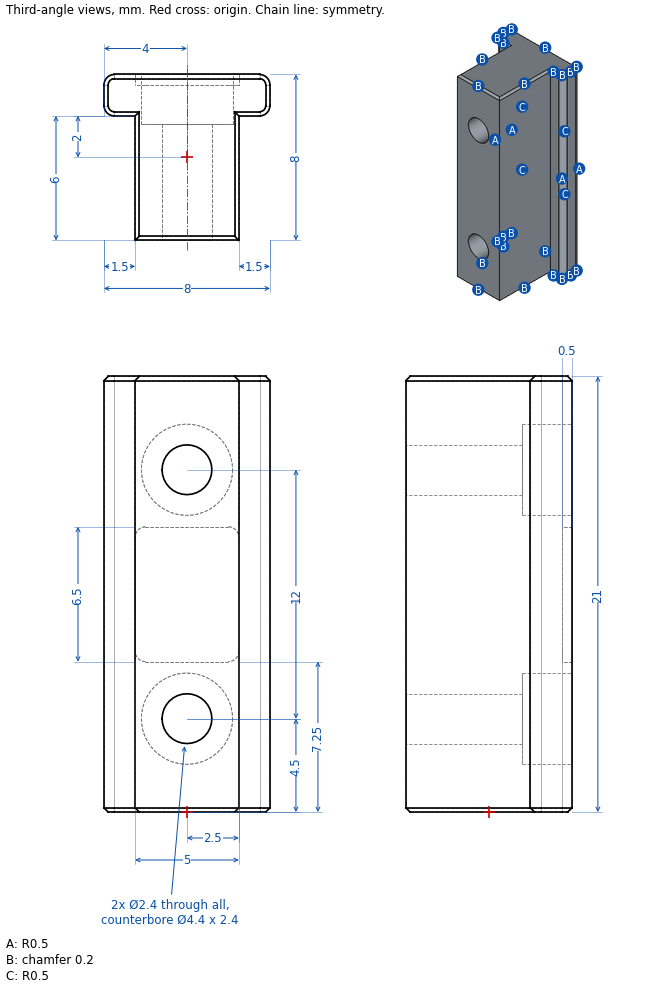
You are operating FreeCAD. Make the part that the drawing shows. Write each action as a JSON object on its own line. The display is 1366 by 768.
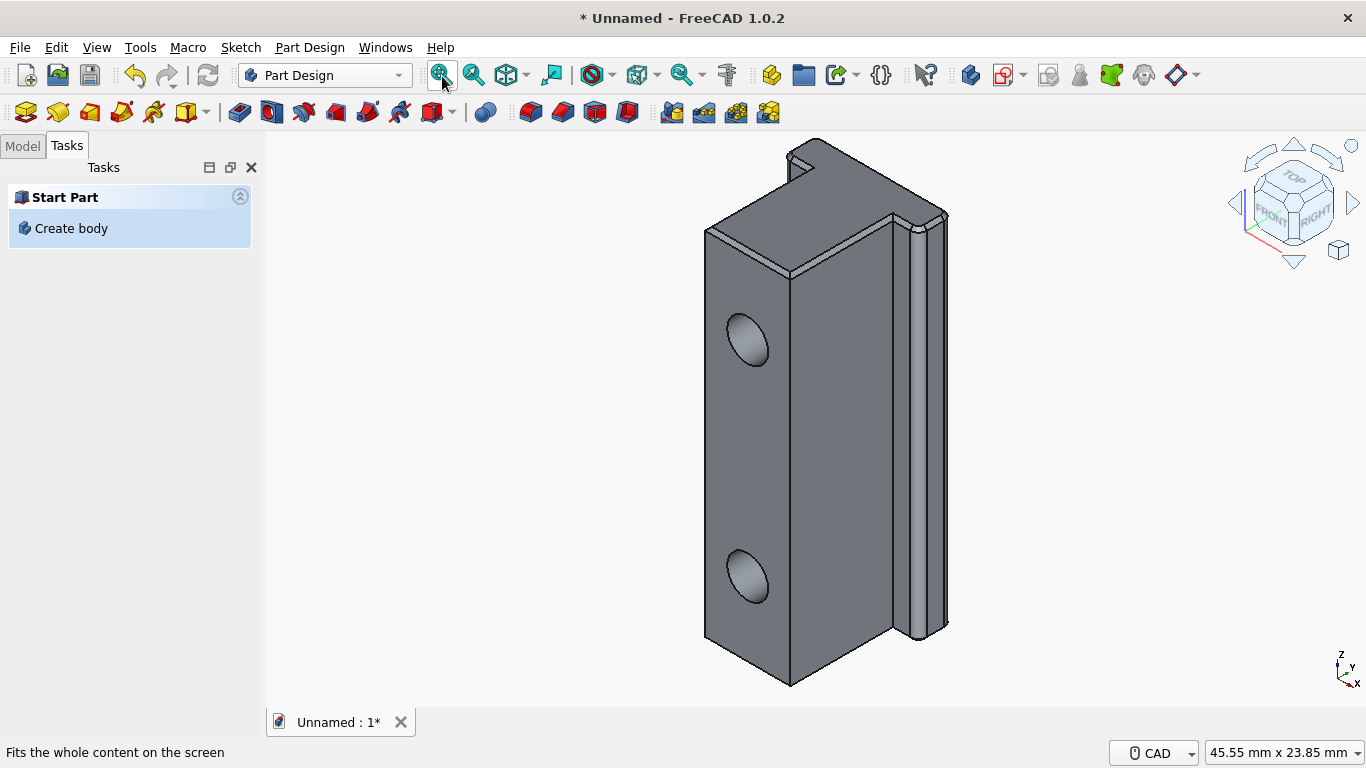
{"action": "key", "text": "2"}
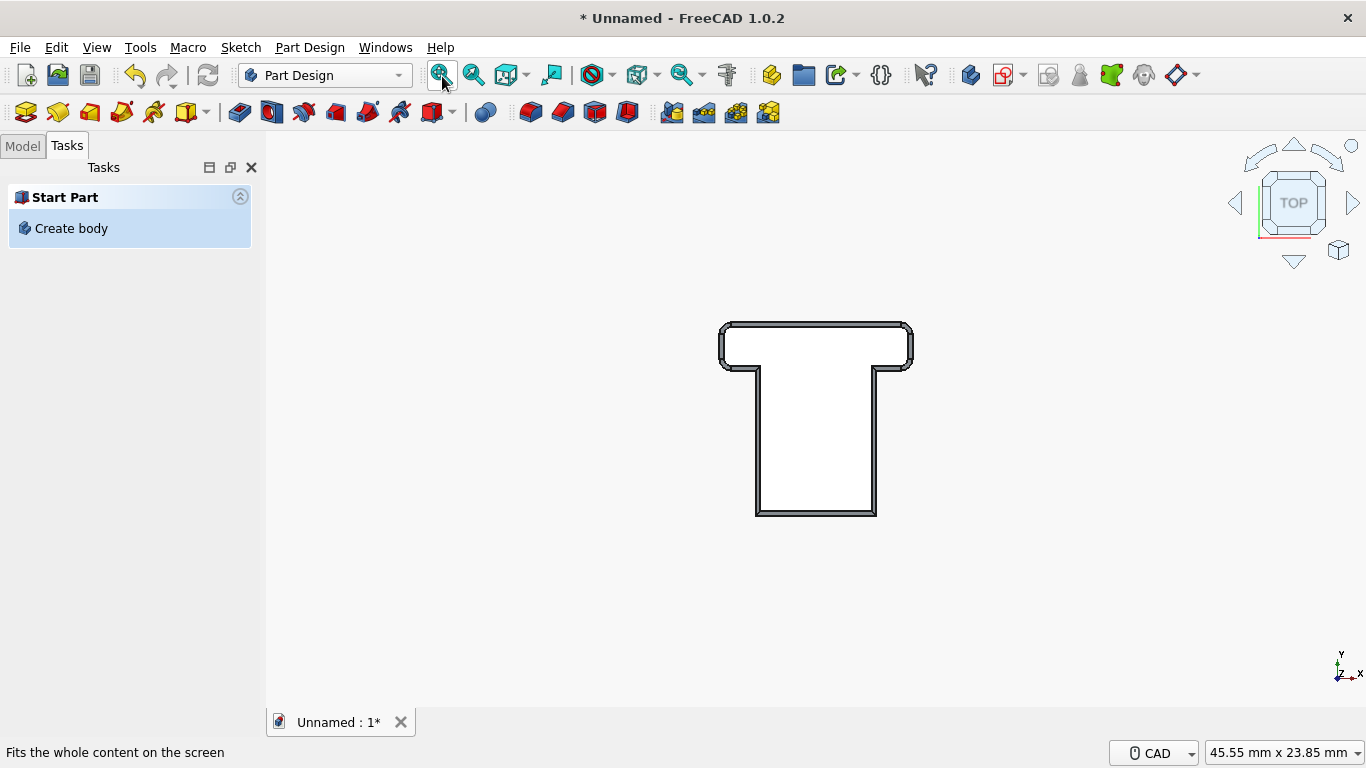
{"action": "left_click", "coordinate": [442, 76]}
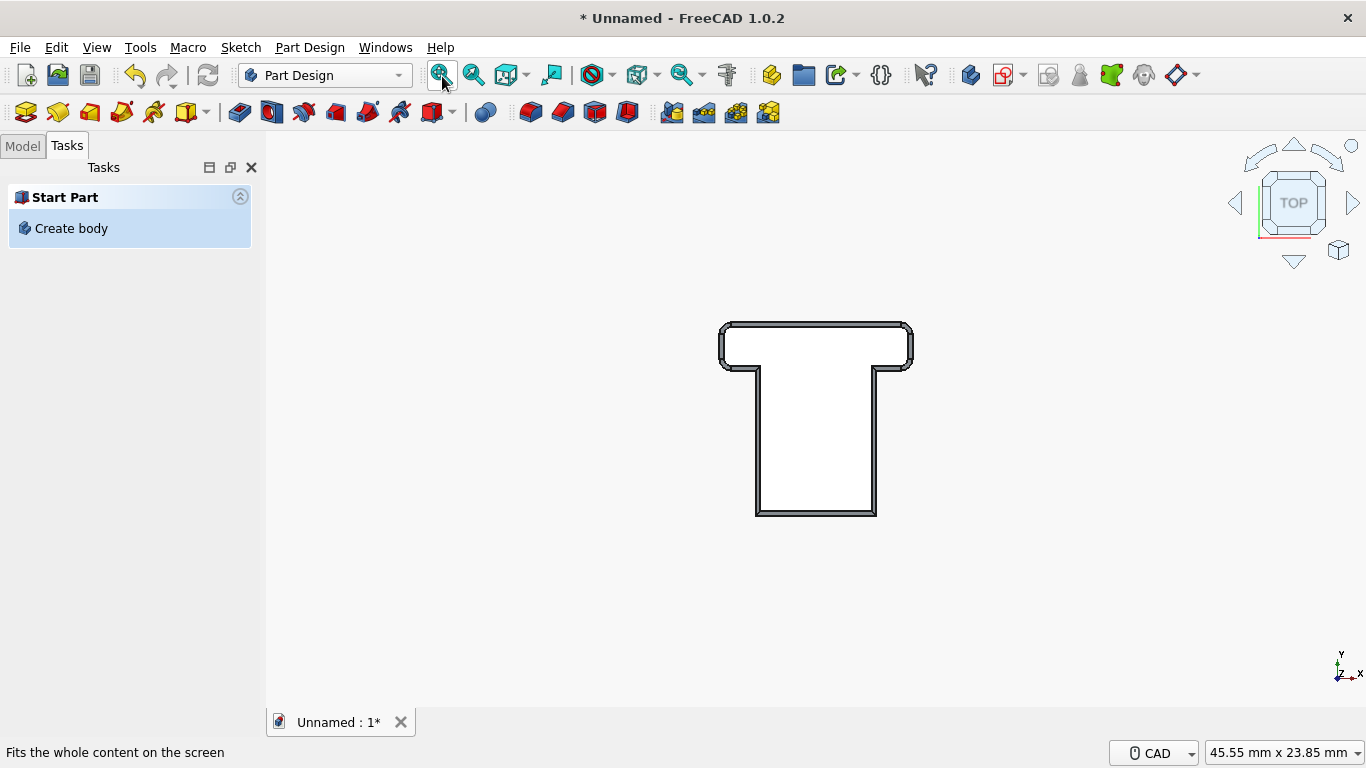
{"action": "scroll", "coordinate": [876, 327], "scroll_direction": "up", "scroll_amount": 6}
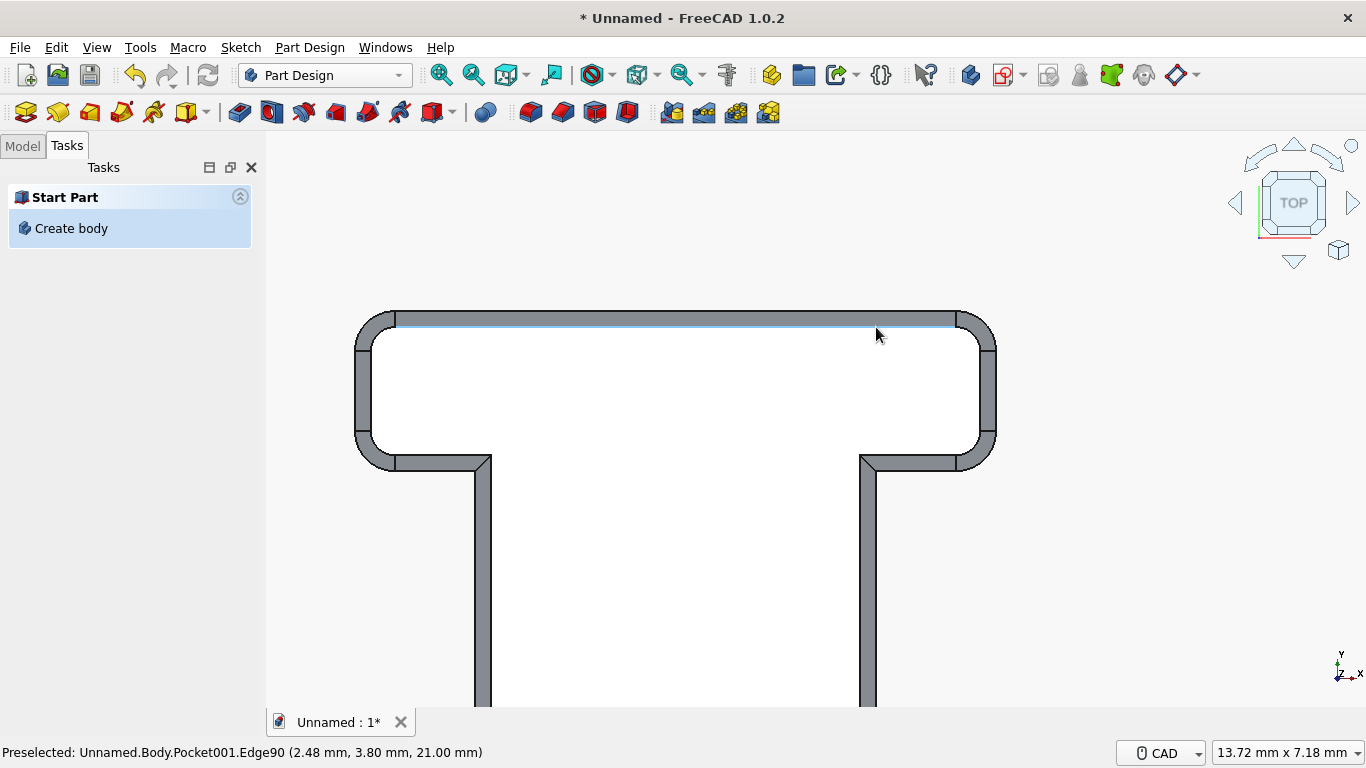
{"action": "left_click", "coordinate": [442, 76]}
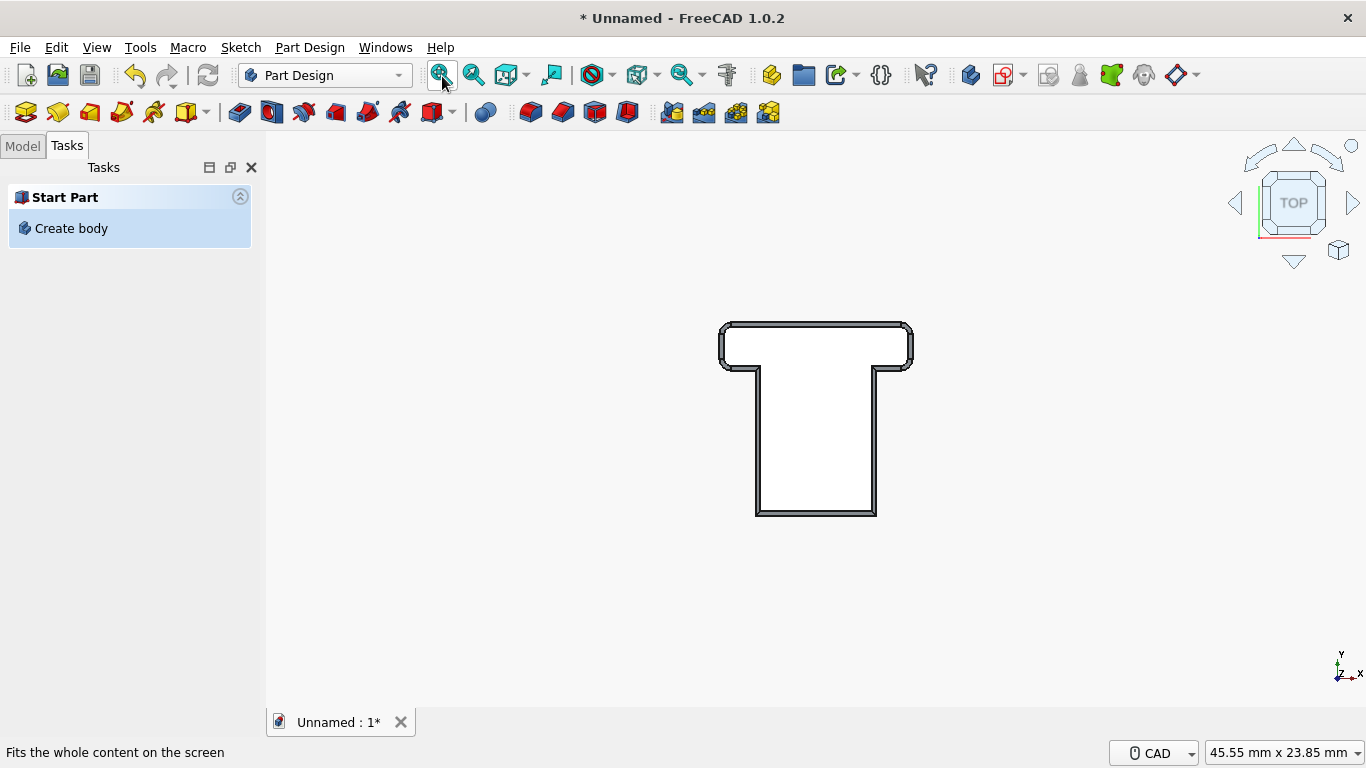
{"action": "key", "text": "1"}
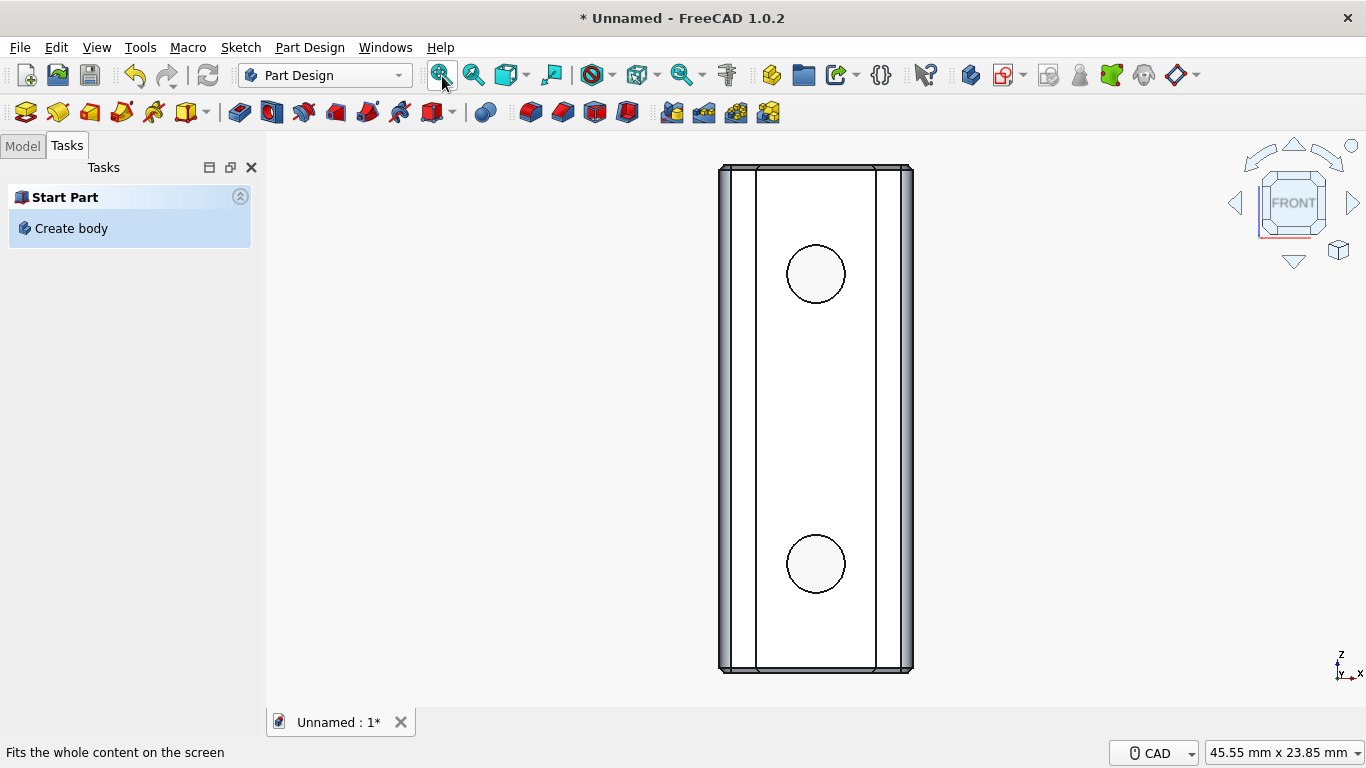
{"action": "scroll", "coordinate": [876, 496], "scroll_direction": "up", "scroll_amount": 6}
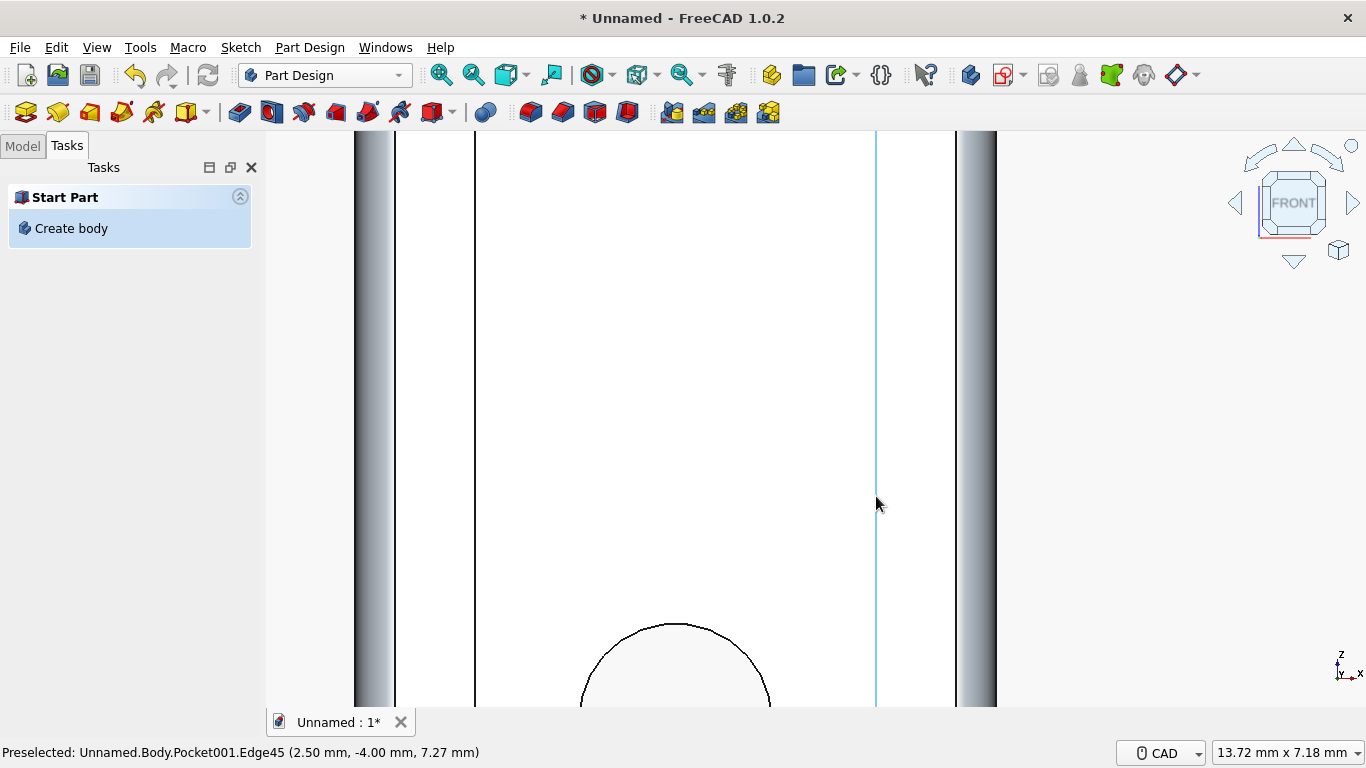
{"action": "left_click", "coordinate": [442, 76]}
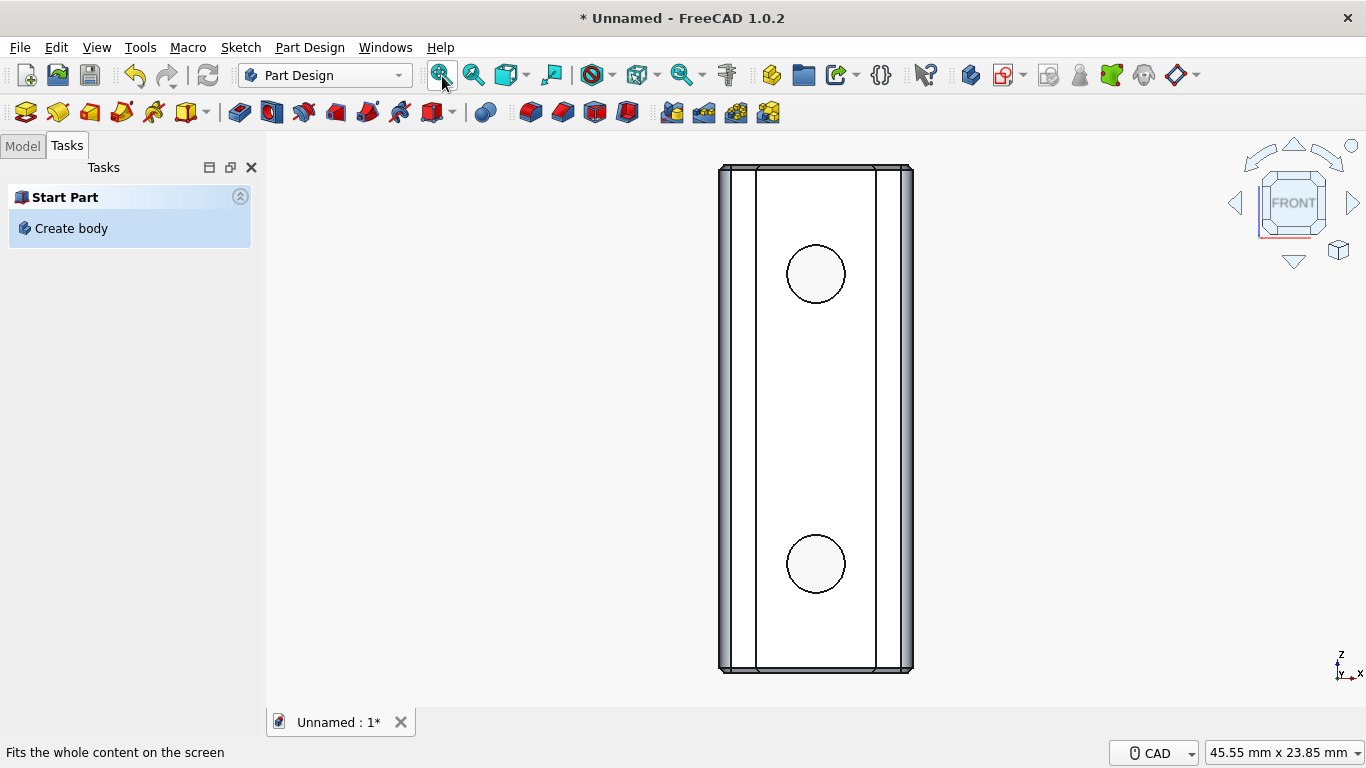
{"action": "key", "text": "3"}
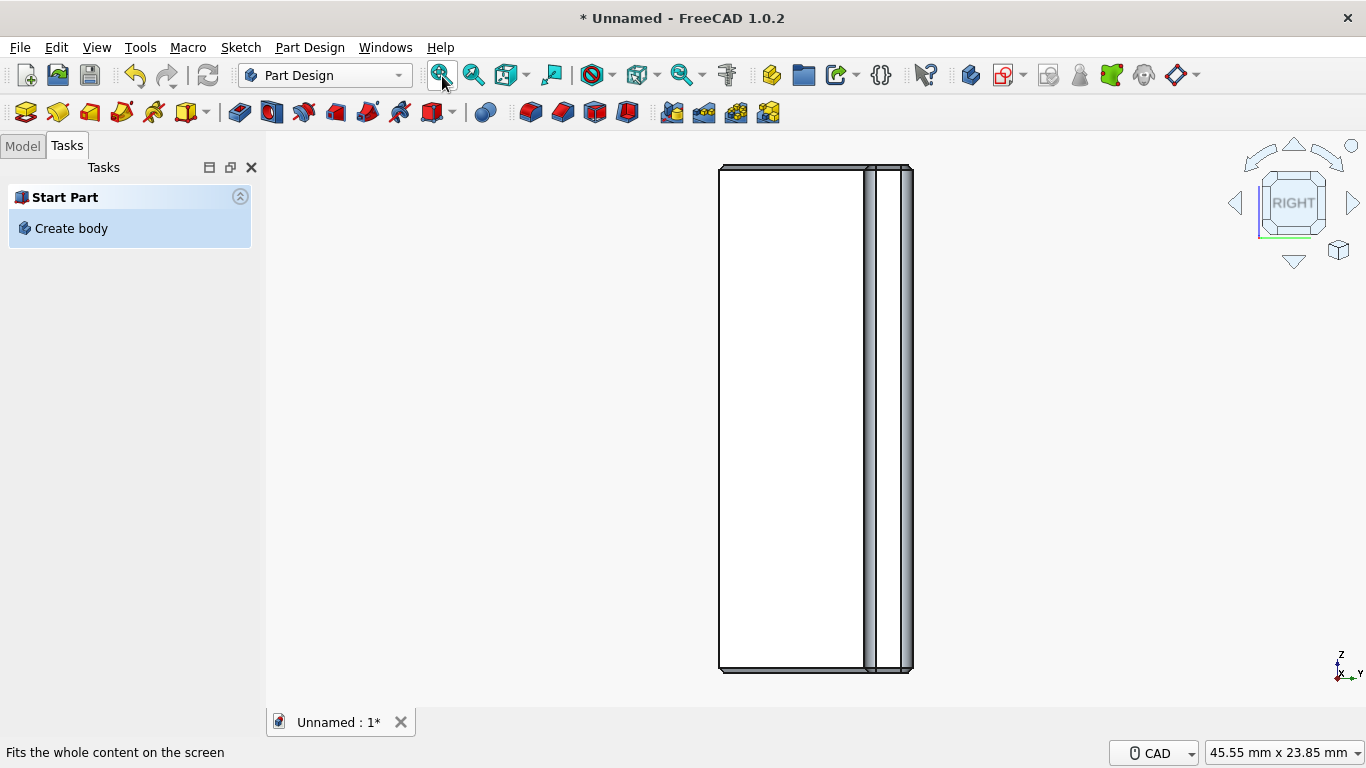
{"action": "scroll", "coordinate": [907, 496], "scroll_direction": "up", "scroll_amount": 6}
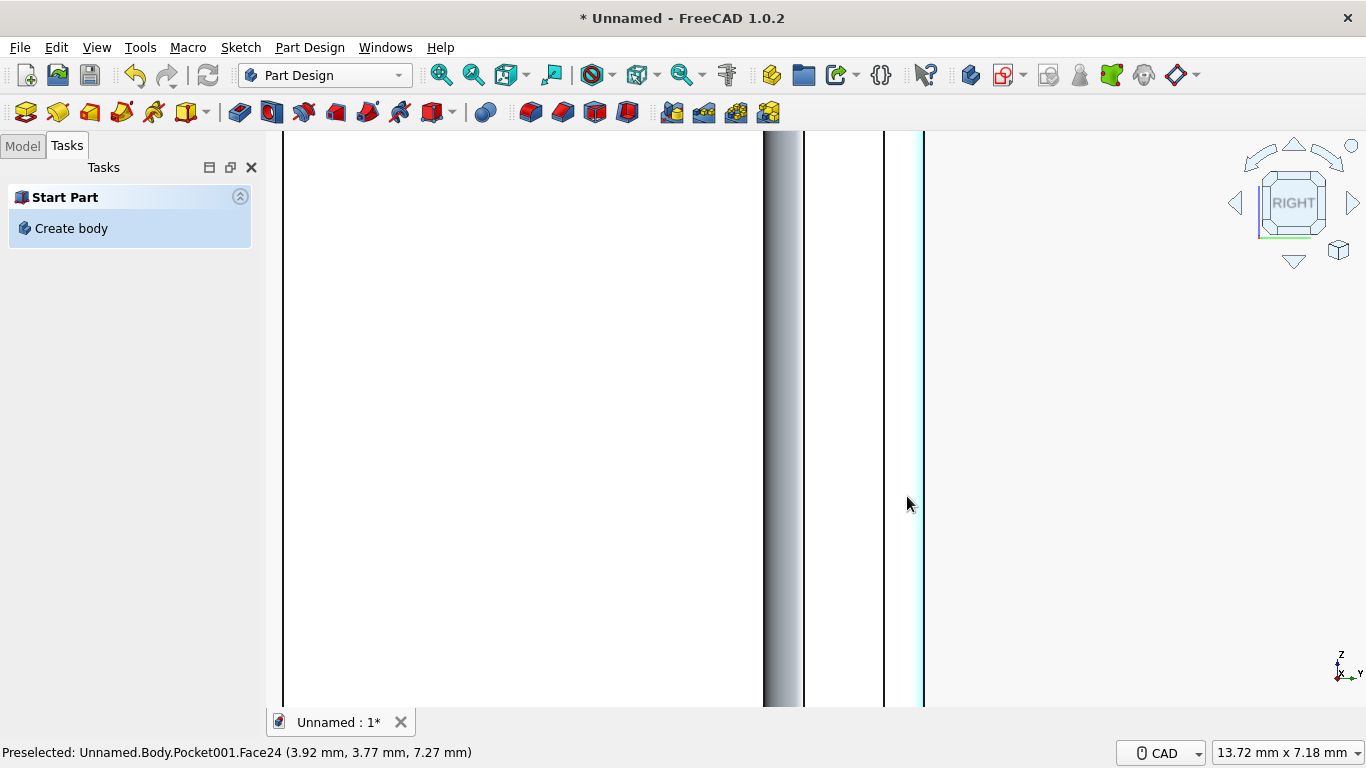
{"action": "left_click", "coordinate": [442, 76]}